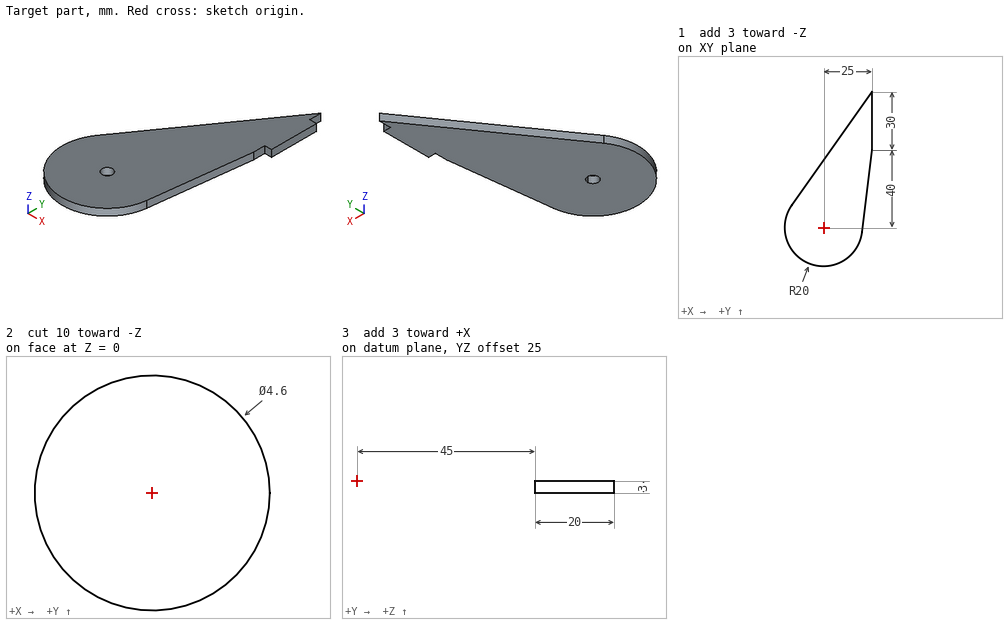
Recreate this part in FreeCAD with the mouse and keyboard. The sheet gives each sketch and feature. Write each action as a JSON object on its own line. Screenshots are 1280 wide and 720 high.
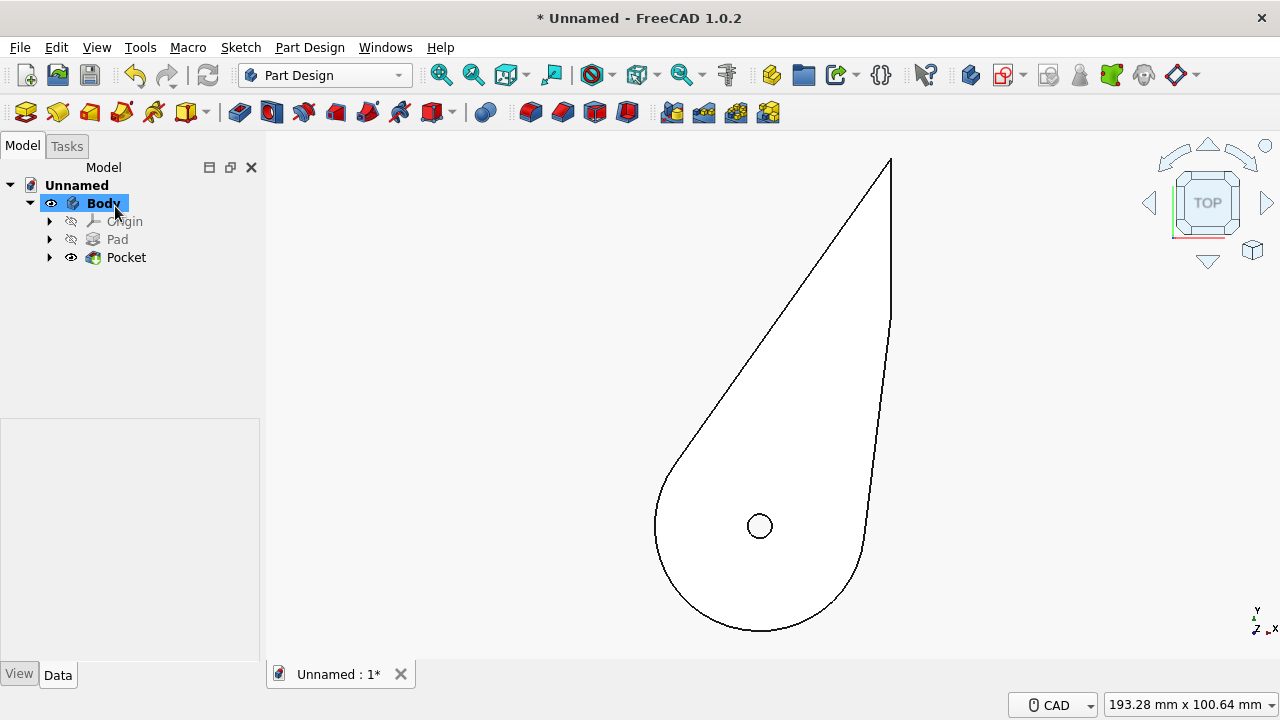
{"action": "left_click", "coordinate": [50, 221]}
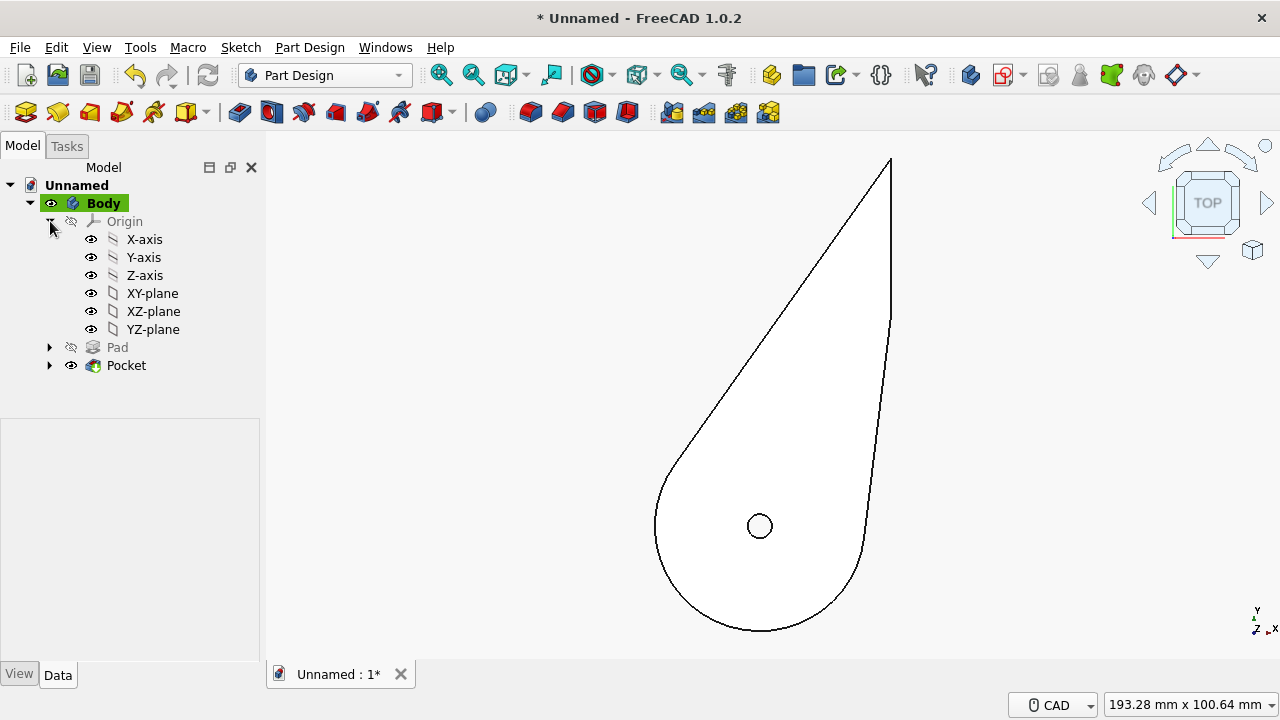
{"action": "left_click", "coordinate": [136, 329]}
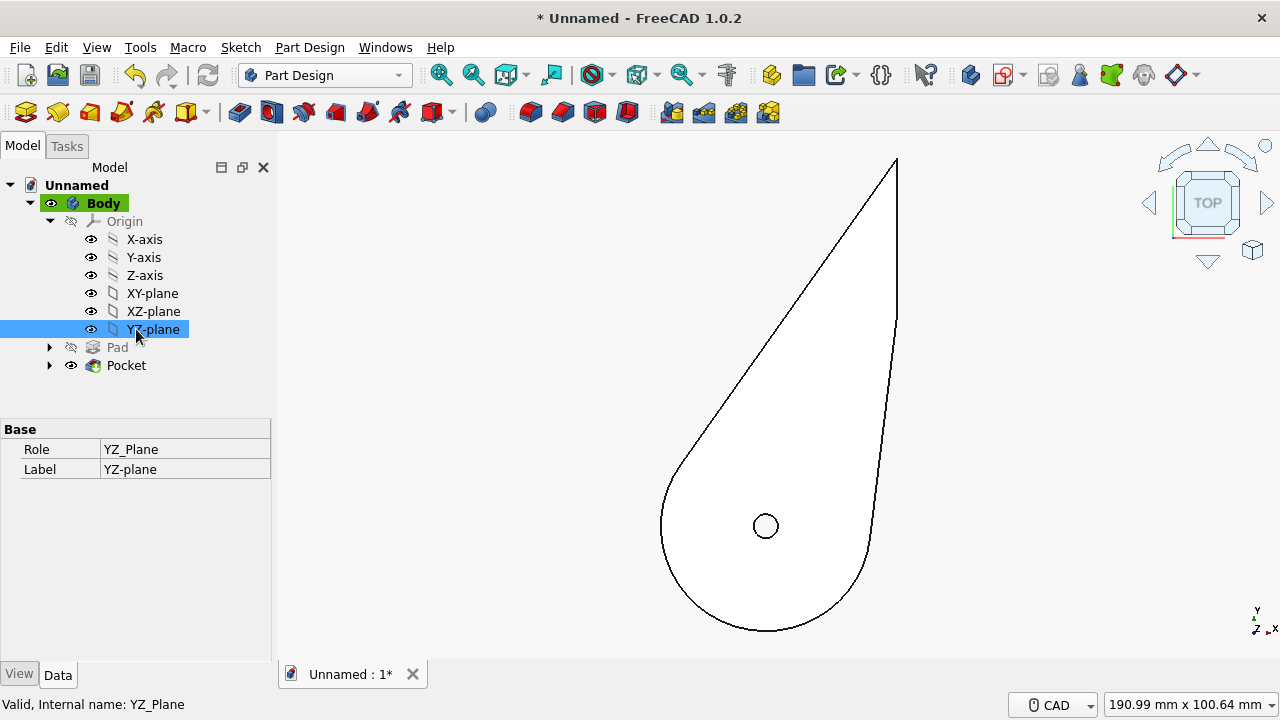
{"action": "left_click", "coordinate": [1176, 76]}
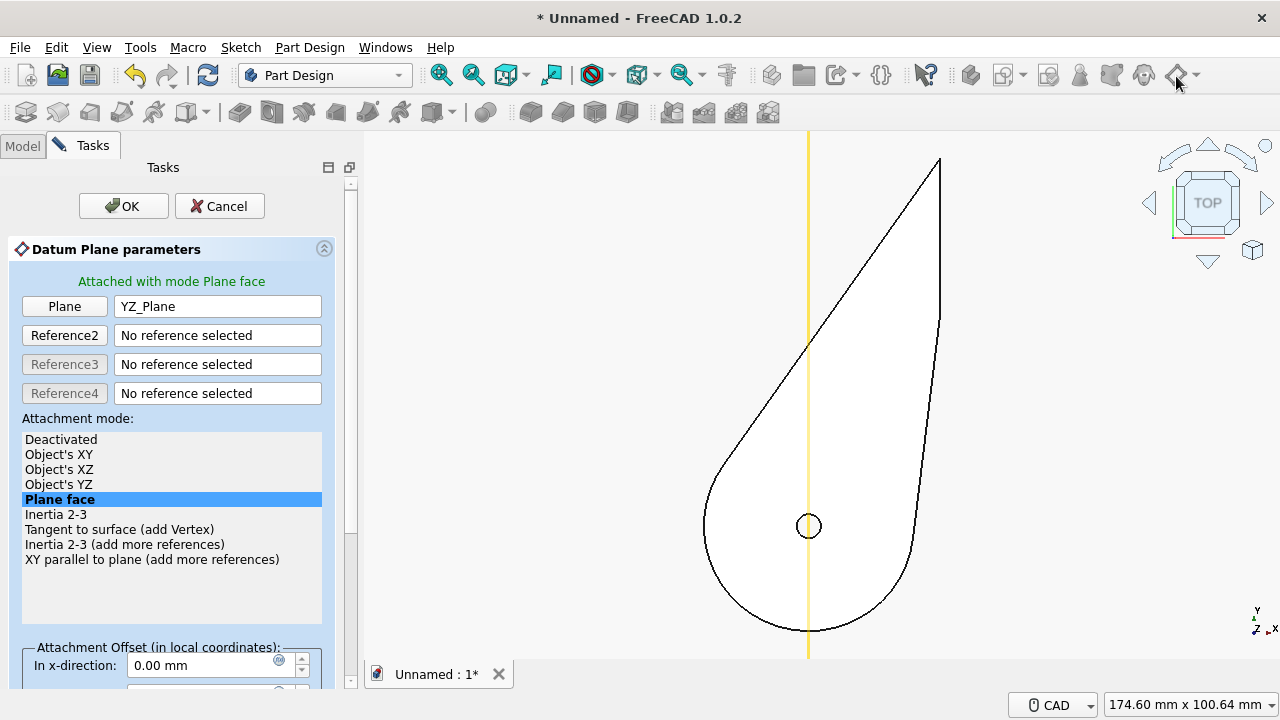
{"action": "scroll", "coordinate": [351, 432], "scroll_direction": "down", "scroll_amount": 2}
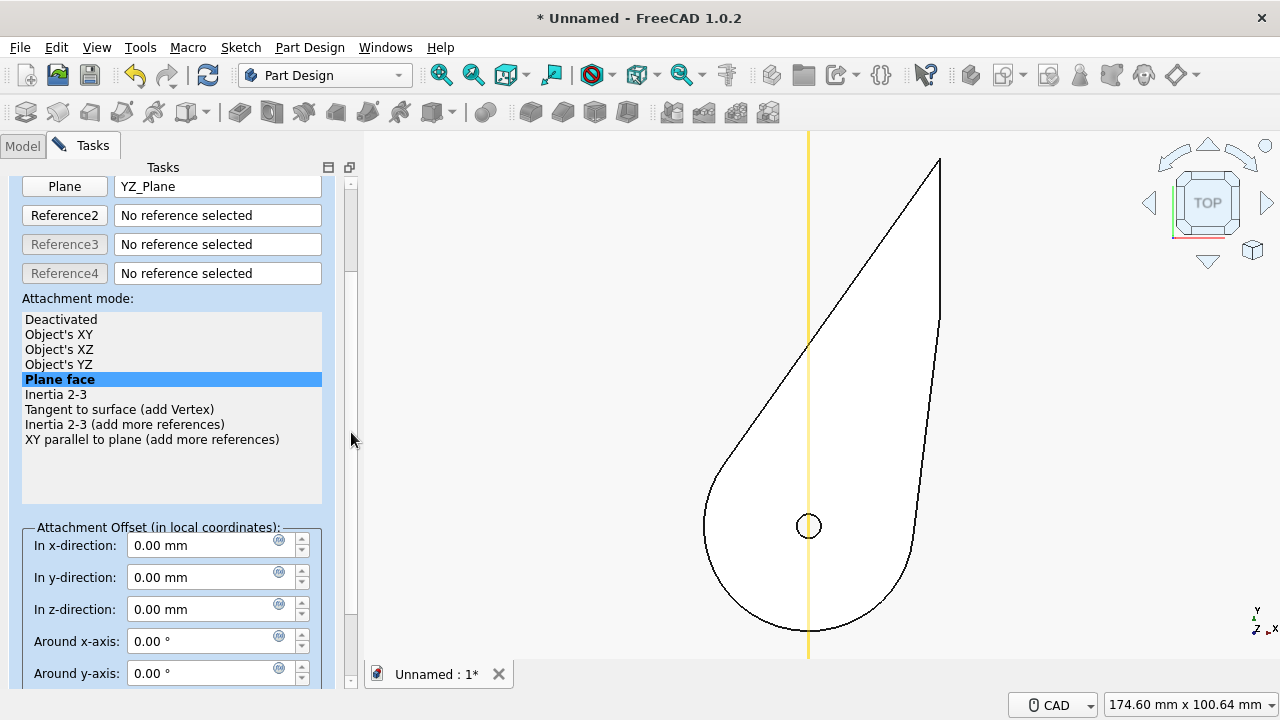
{"action": "triple_click", "coordinate": [210, 609]}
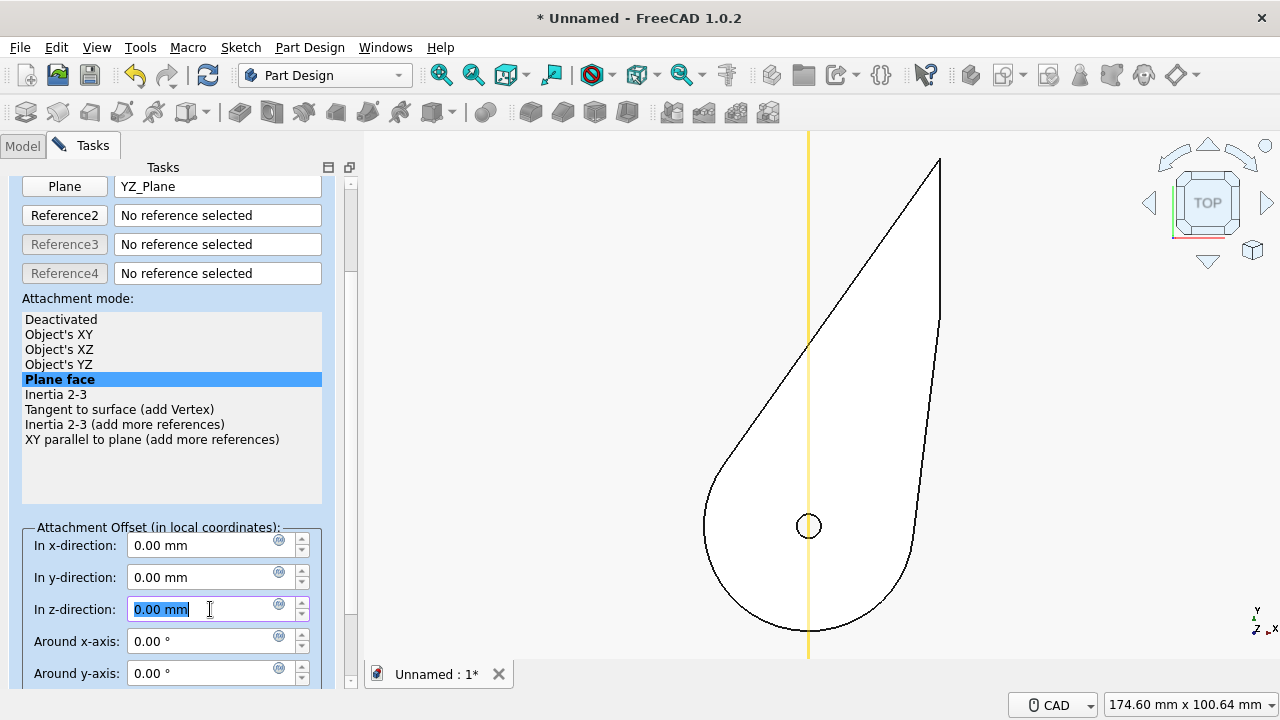
{"action": "type", "text": "25"}
{"action": "key", "text": "Tab"}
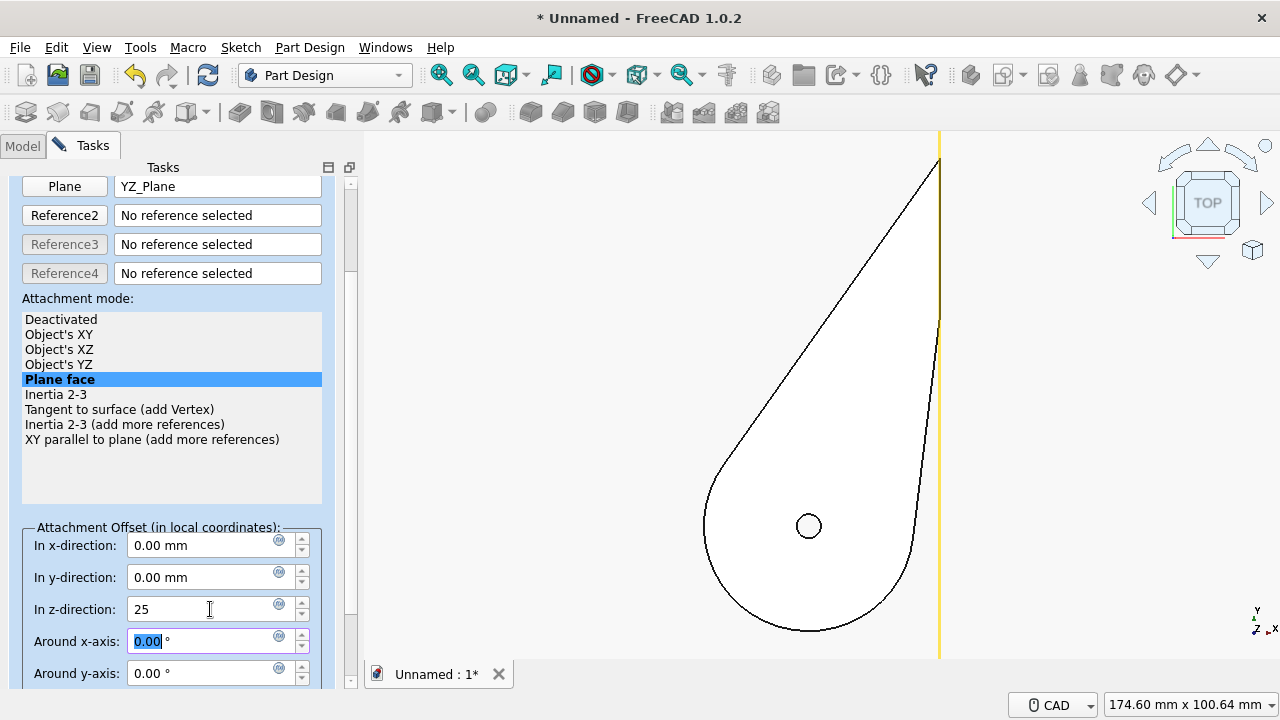
{"action": "scroll", "coordinate": [351, 432], "scroll_direction": "up", "scroll_amount": 3}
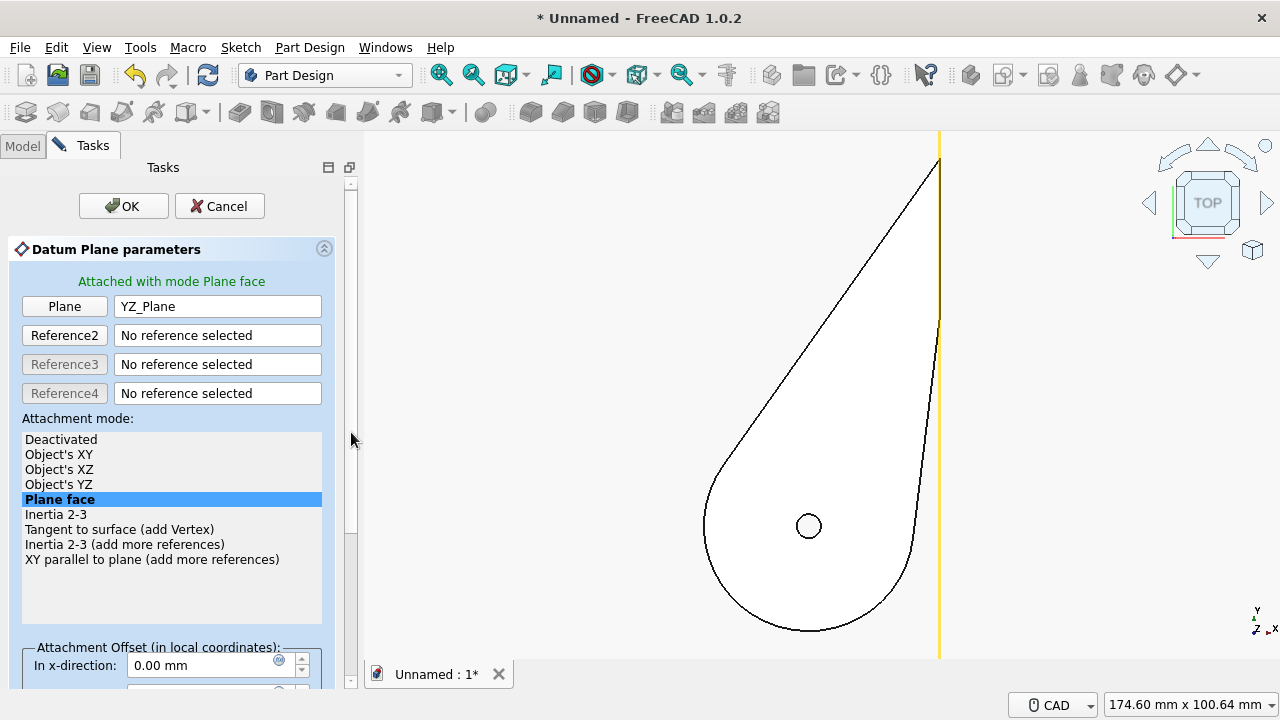
{"action": "left_click", "coordinate": [124, 206]}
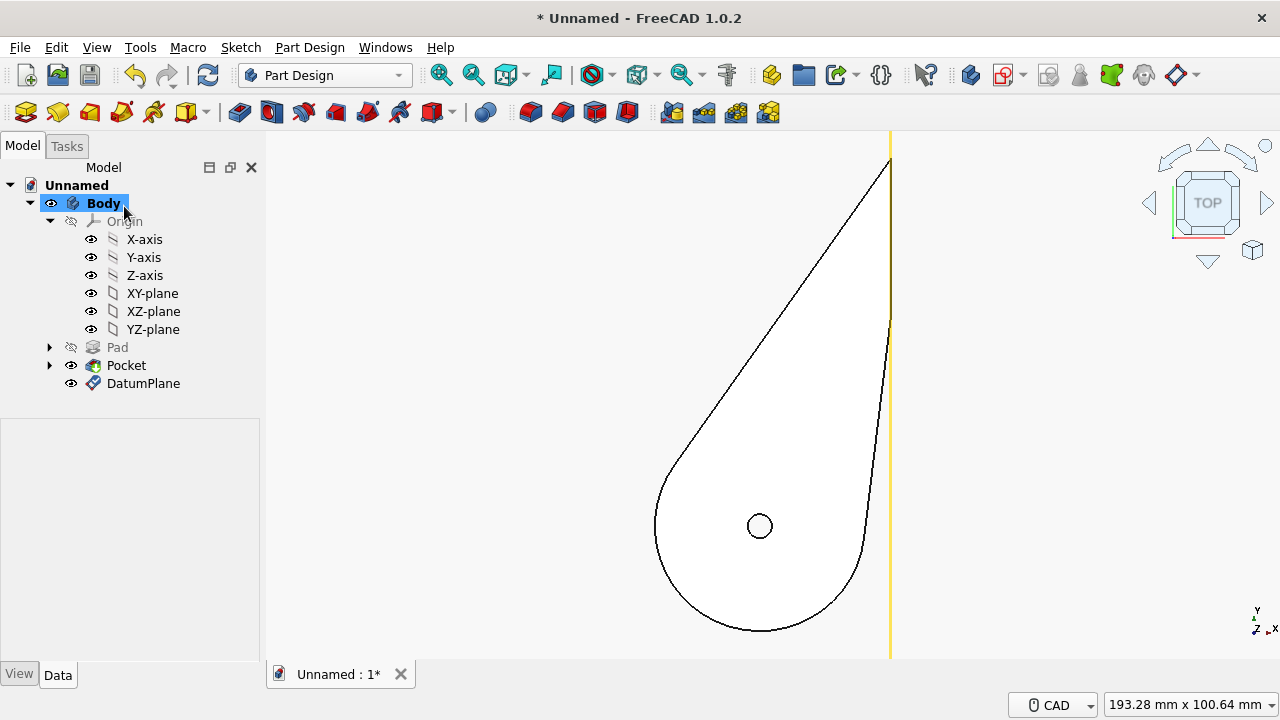
{"action": "left_click", "coordinate": [116, 383]}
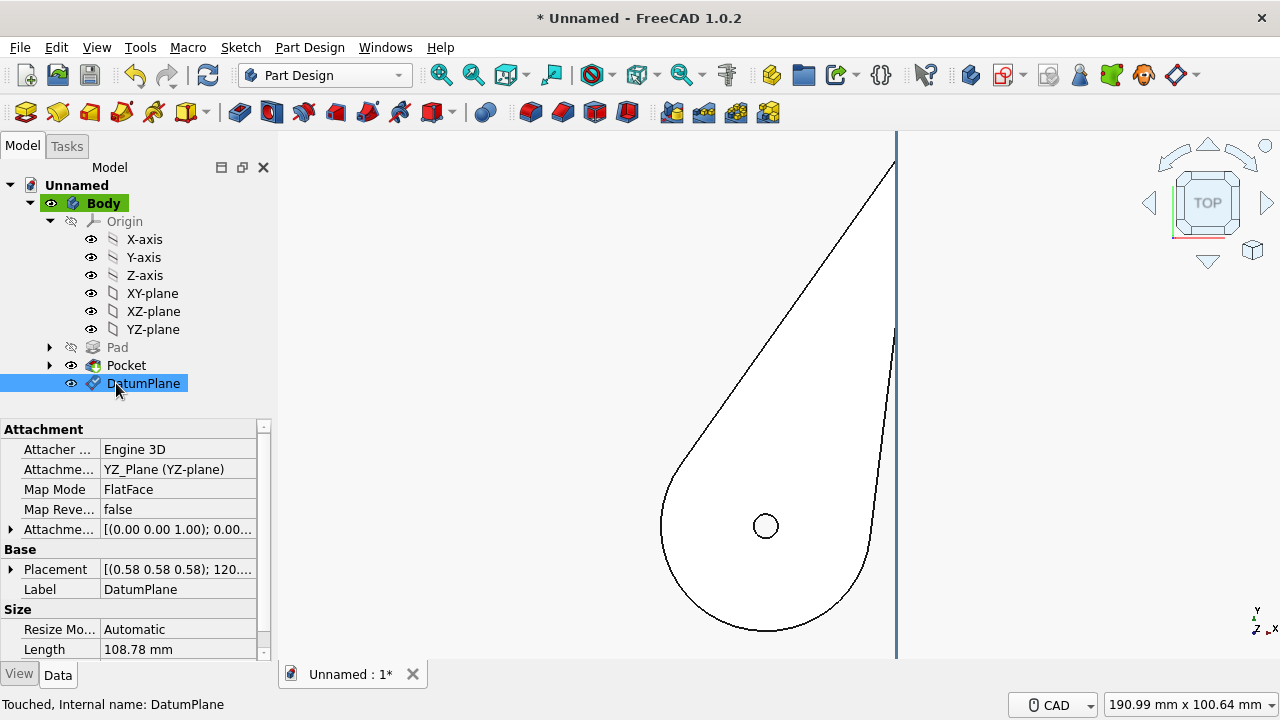
{"action": "left_click", "coordinate": [1004, 76]}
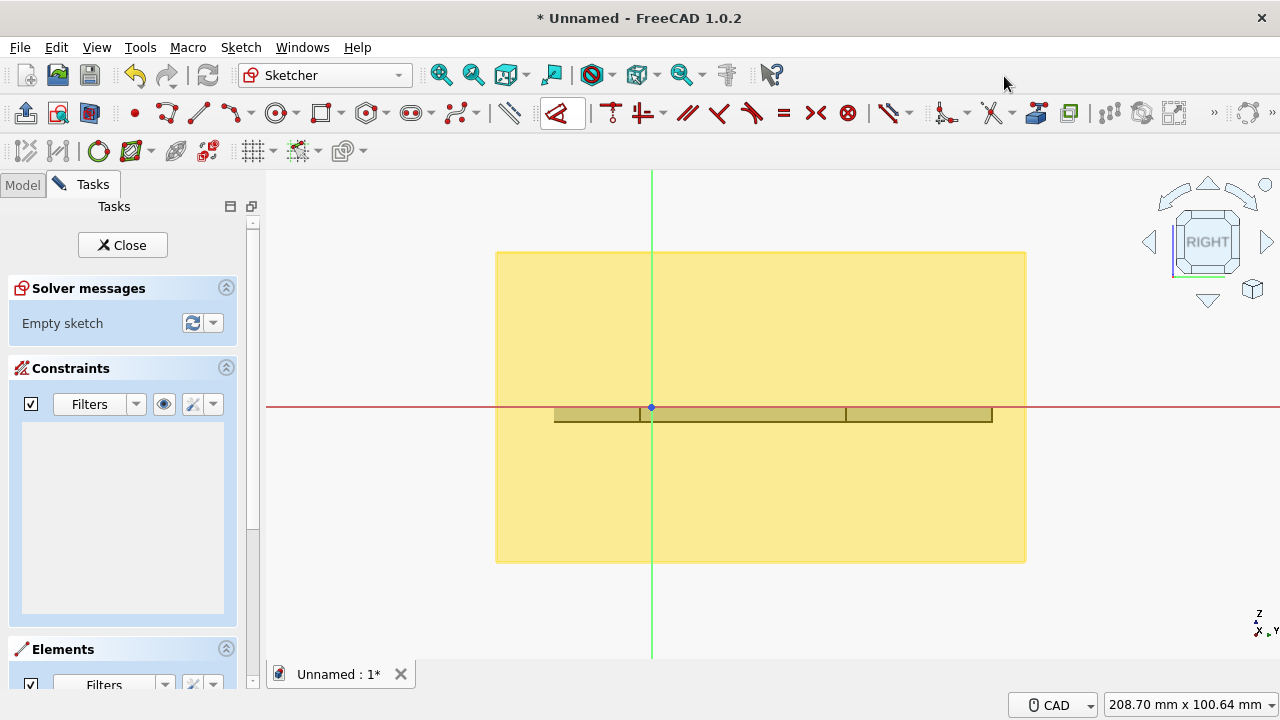
{"action": "scroll", "coordinate": [961, 414], "scroll_direction": "up", "scroll_amount": 9}